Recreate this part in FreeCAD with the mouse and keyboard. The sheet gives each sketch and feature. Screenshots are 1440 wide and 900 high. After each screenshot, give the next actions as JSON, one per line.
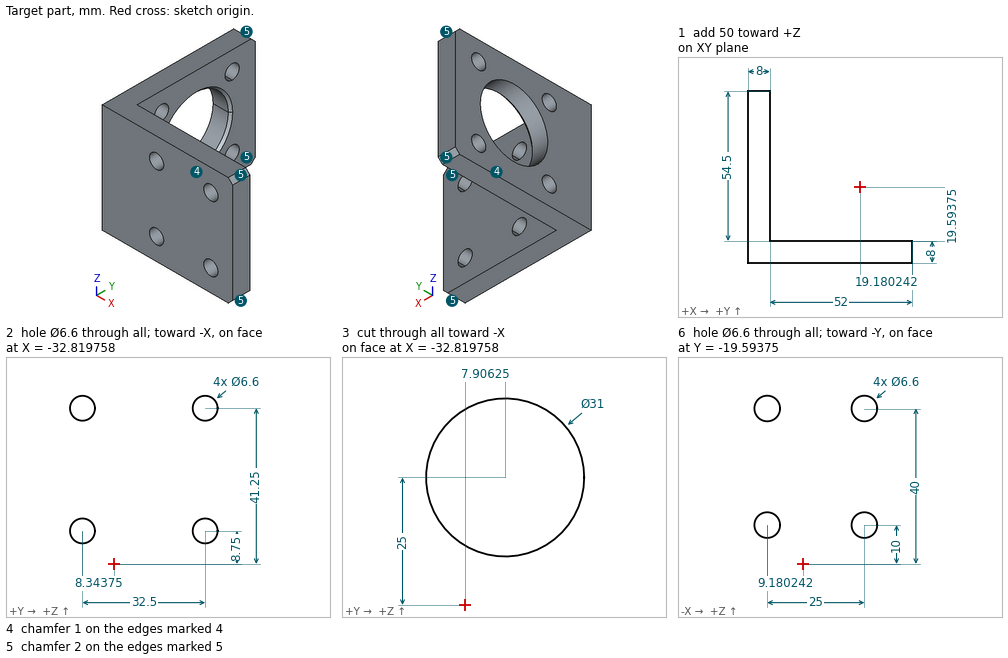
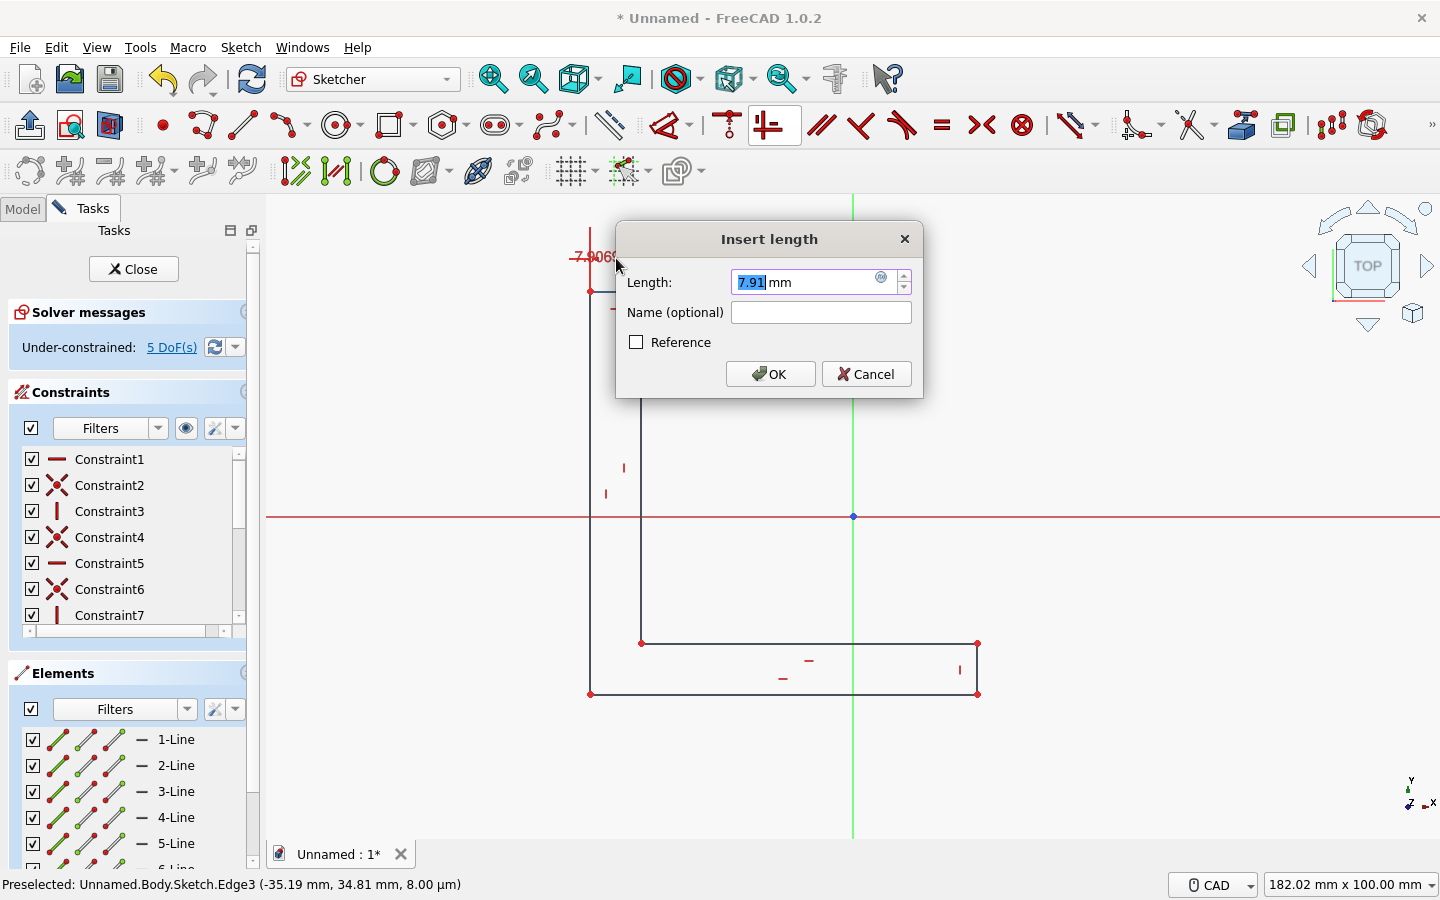
{"action": "type", "text": "8"}
{"action": "key", "text": "Return"}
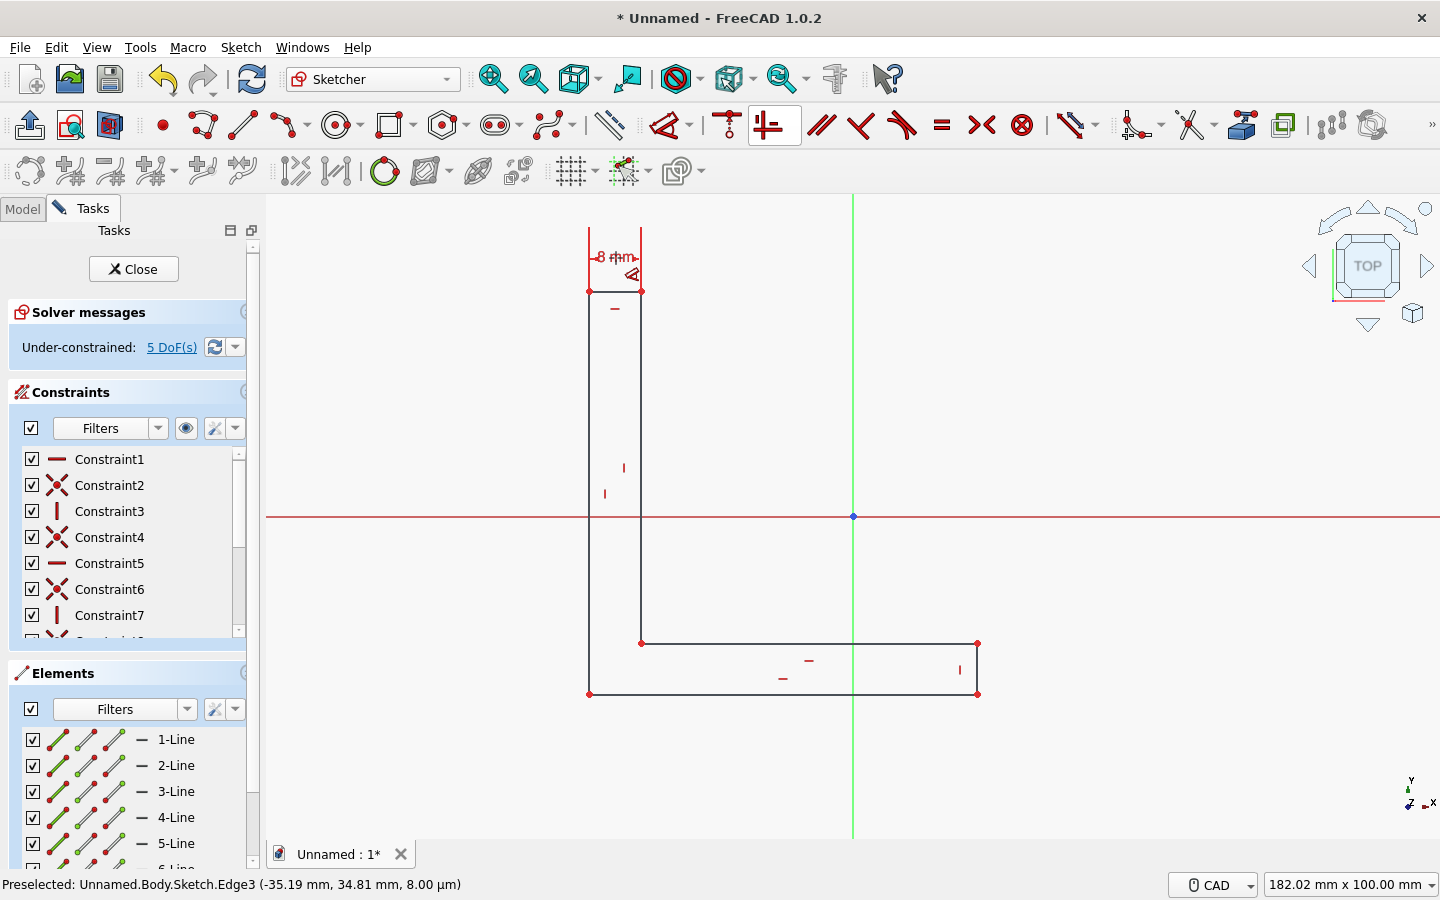
{"action": "left_click", "coordinate": [977, 680]}
{"action": "left_click", "coordinate": [1011, 670]}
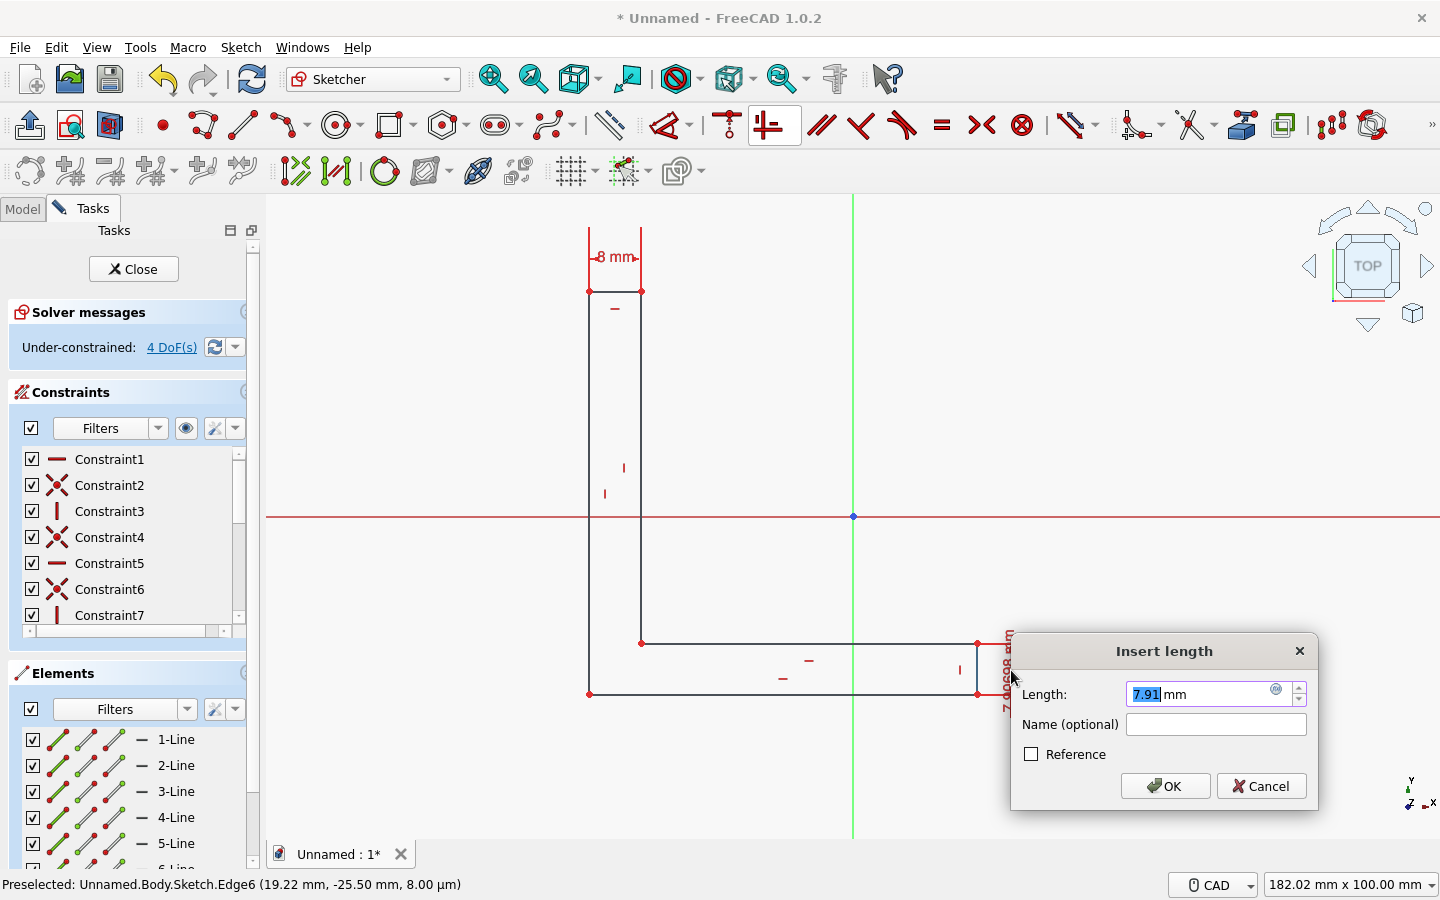
{"action": "type", "text": "8"}
{"action": "key", "text": "Return"}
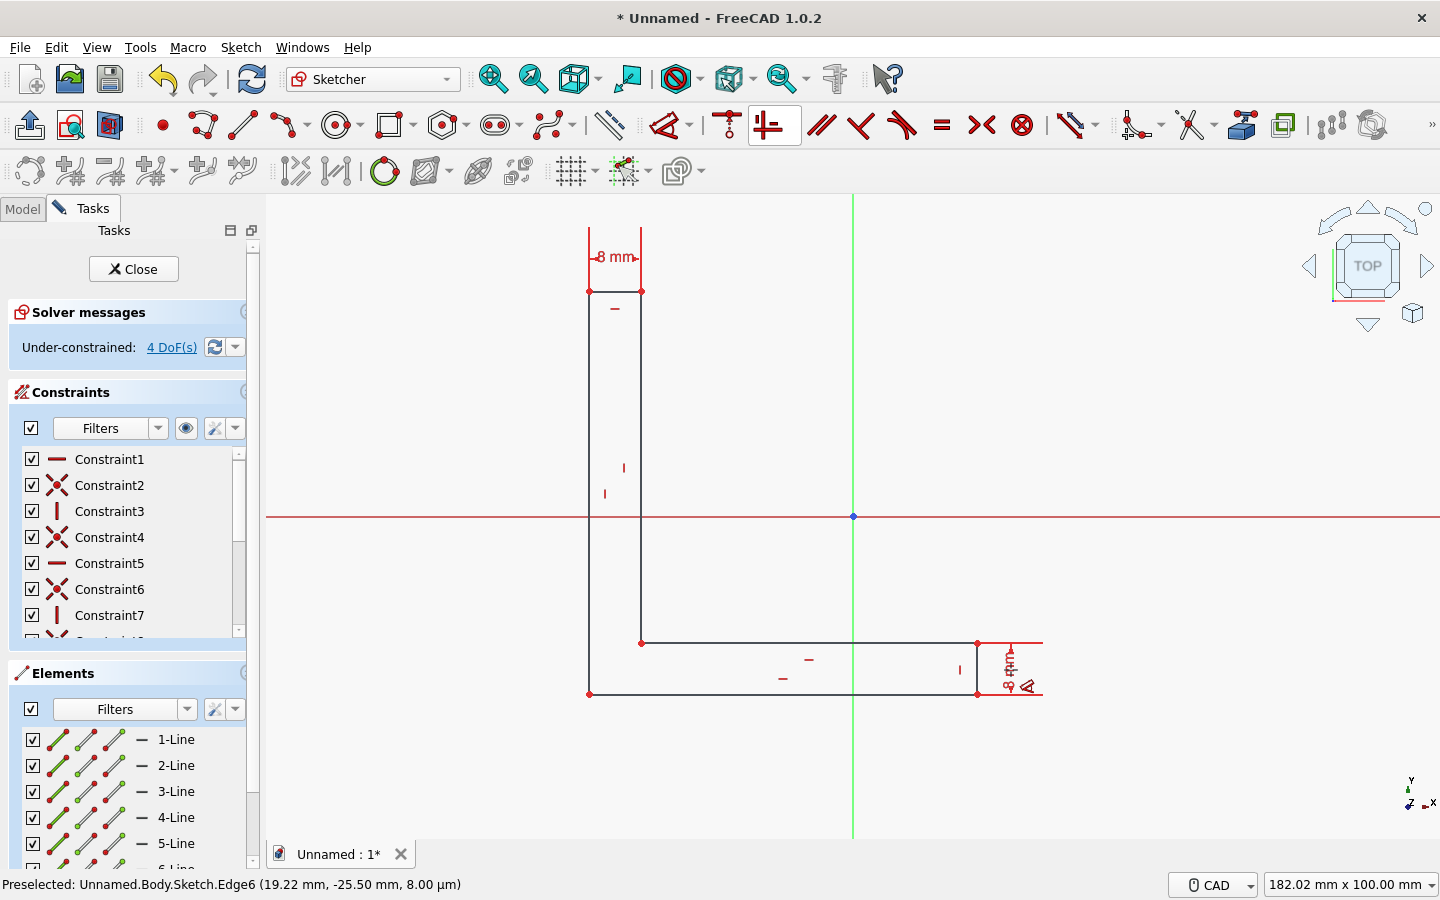
{"action": "left_click", "coordinate": [876, 643]}
{"action": "left_click", "coordinate": [809, 677]}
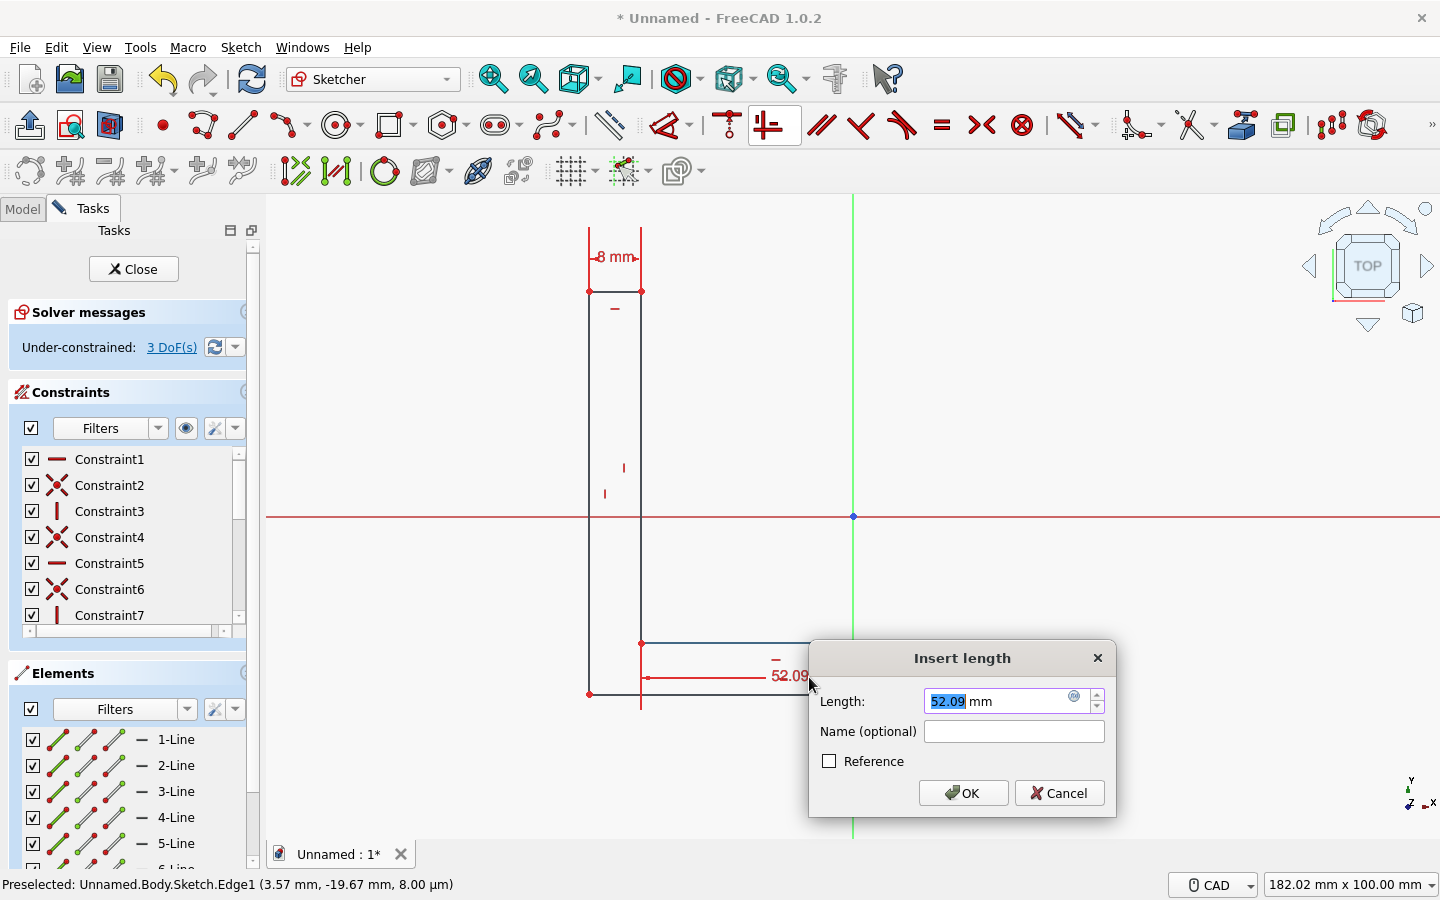
{"action": "type", "text": "52"}
{"action": "key", "text": "Return"}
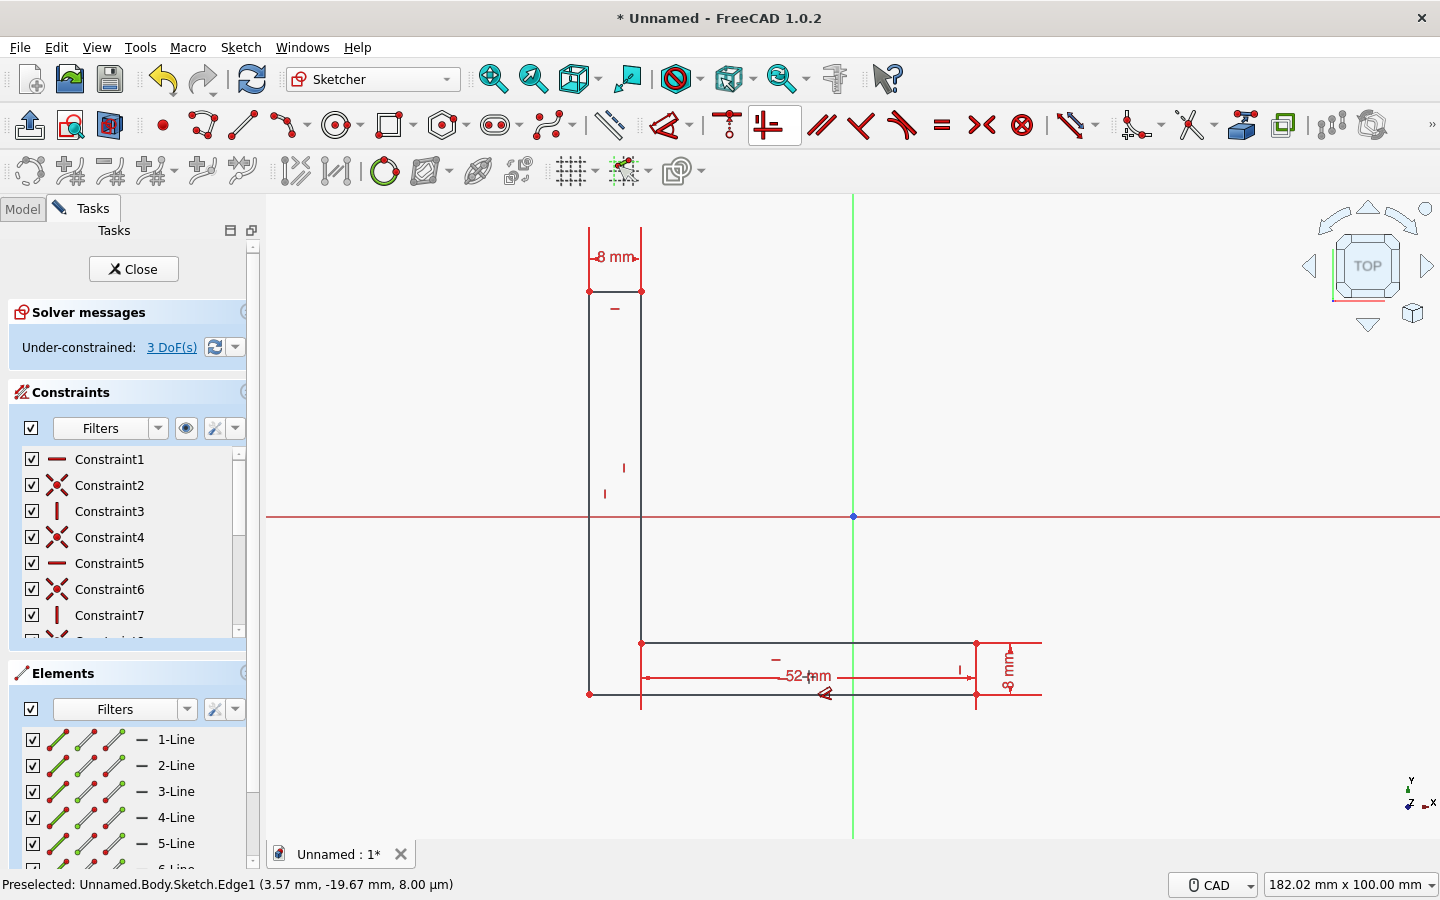
{"action": "left_click", "coordinate": [641, 538]}
{"action": "left_click", "coordinate": [607, 468]}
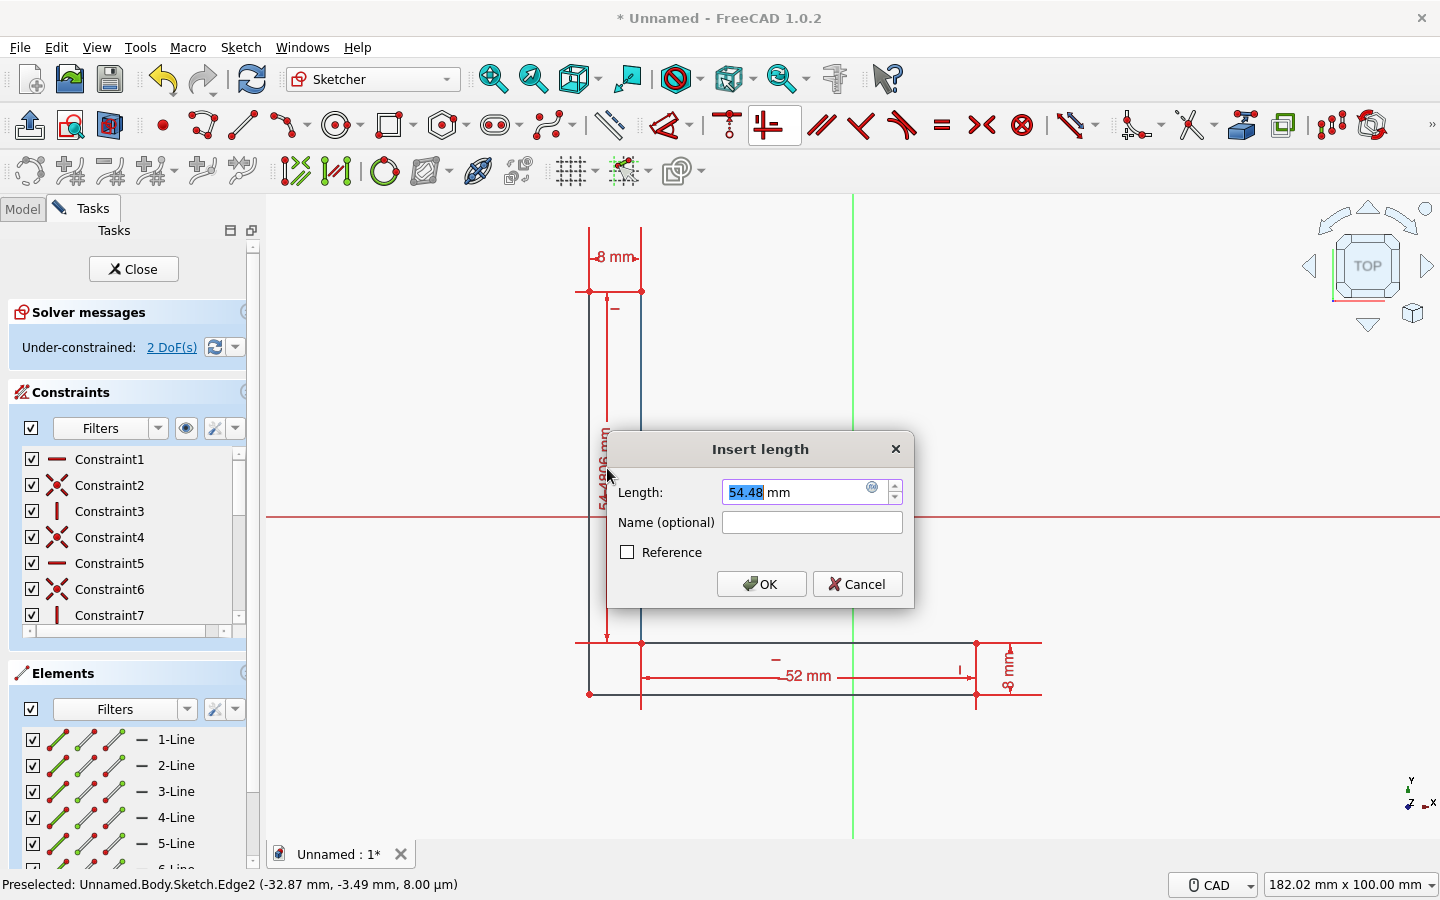
{"action": "type", "text": "54.5"}
{"action": "key", "text": "Return"}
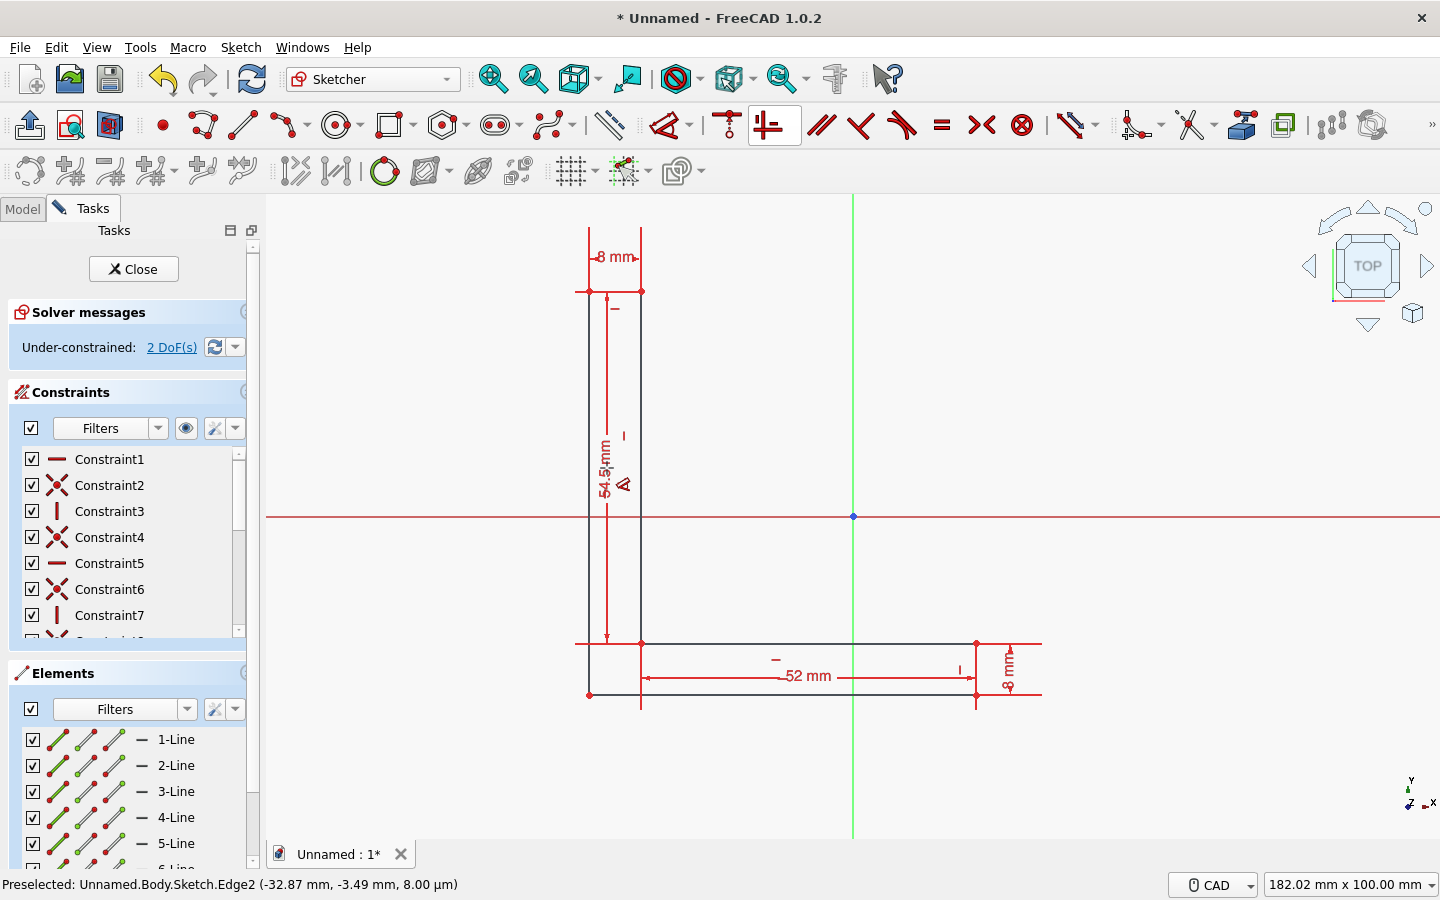
{"action": "left_click", "coordinate": [976, 644]}
{"action": "left_click", "coordinate": [1010, 580]}